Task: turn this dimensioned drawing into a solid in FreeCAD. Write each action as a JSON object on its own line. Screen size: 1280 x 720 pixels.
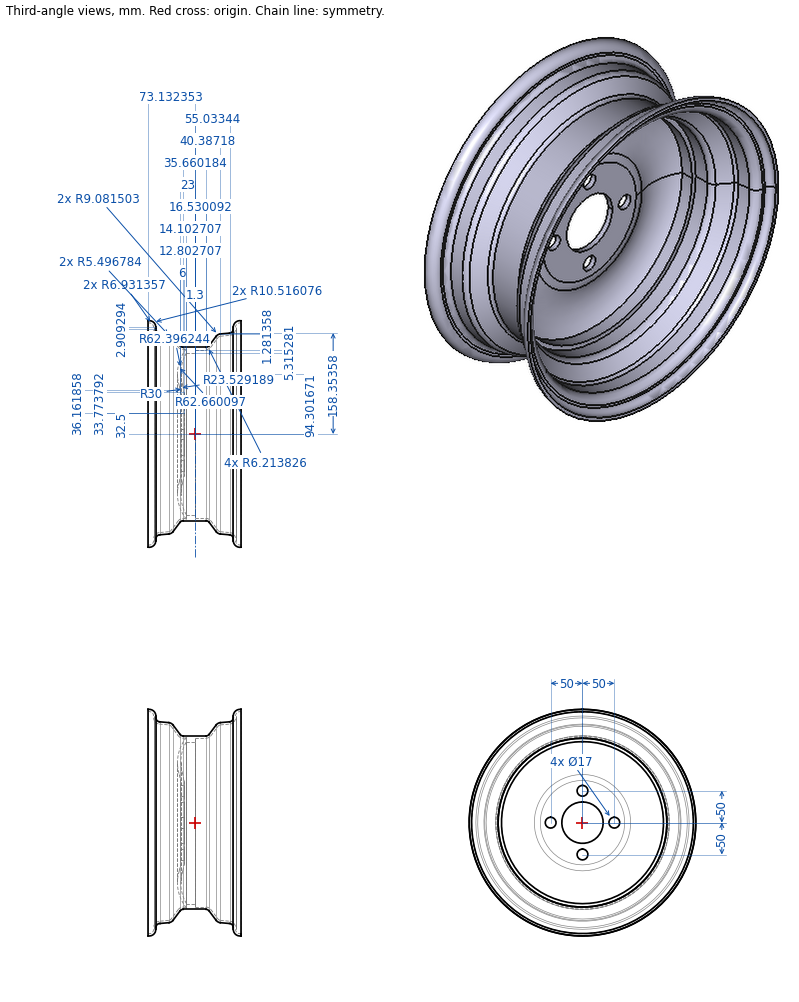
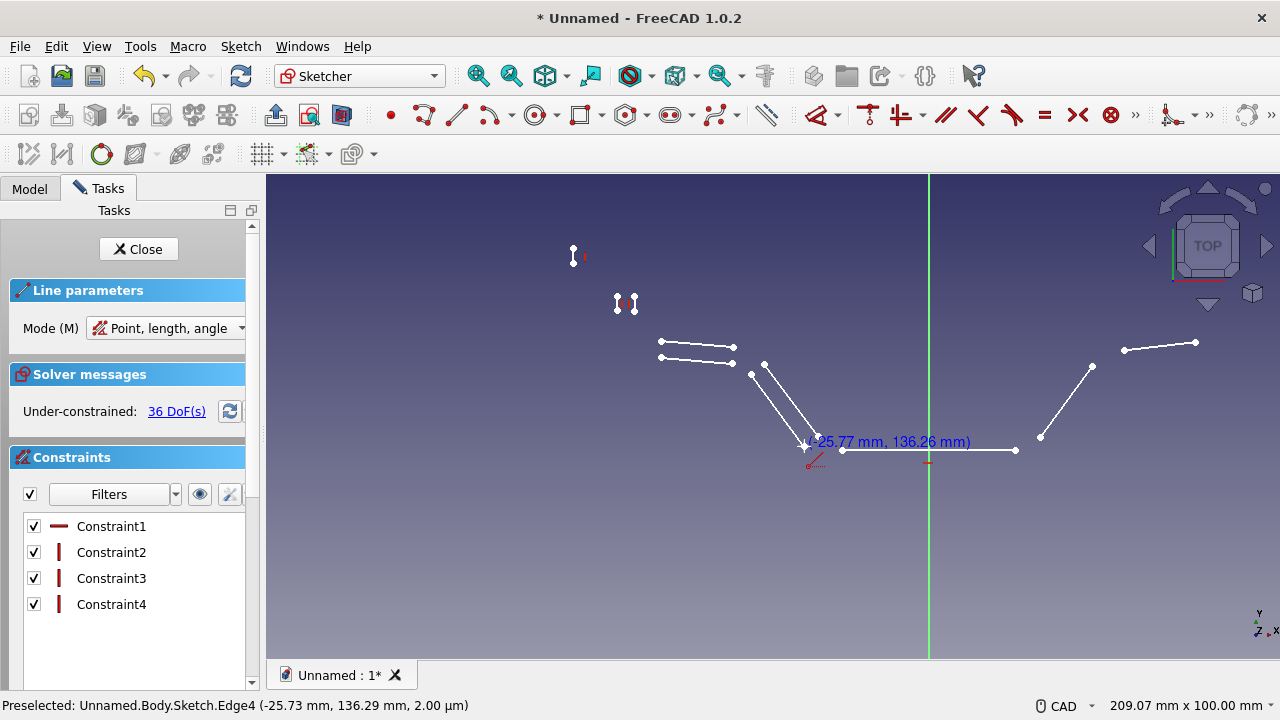
{"action": "key", "text": "g m"}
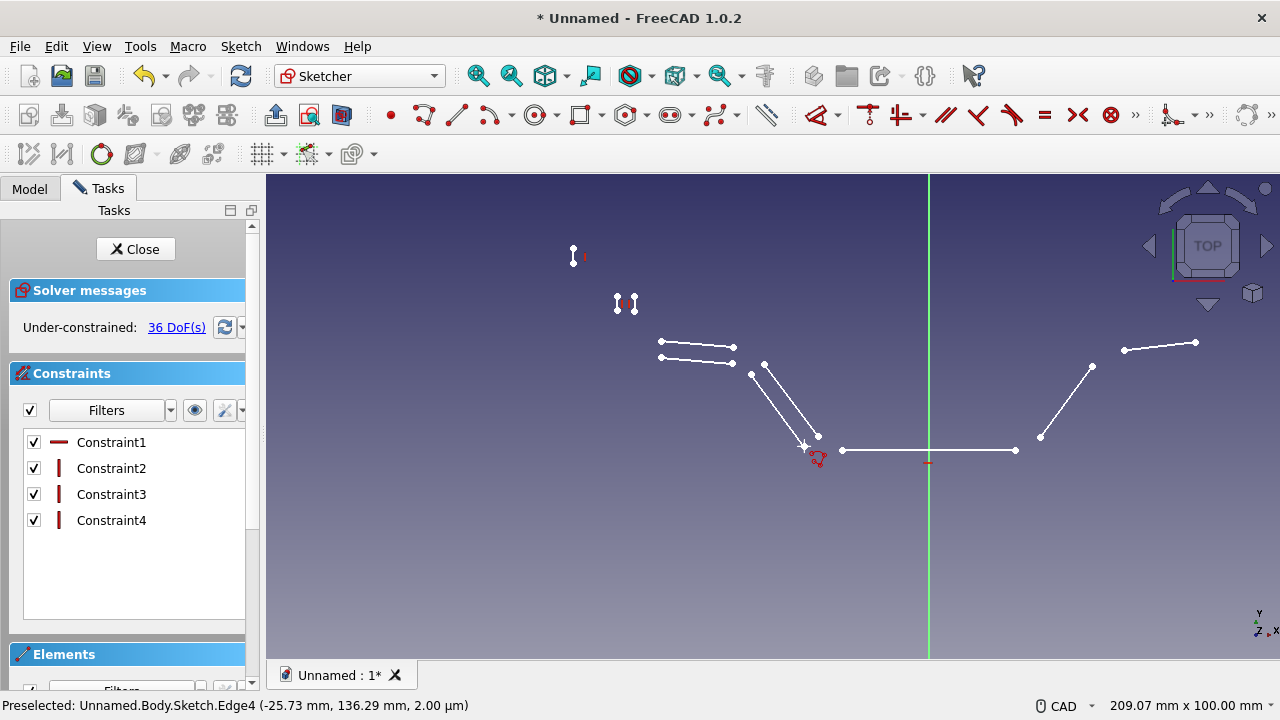
{"action": "scroll", "coordinate": [574, 265], "scroll_direction": "down", "scroll_amount": 5}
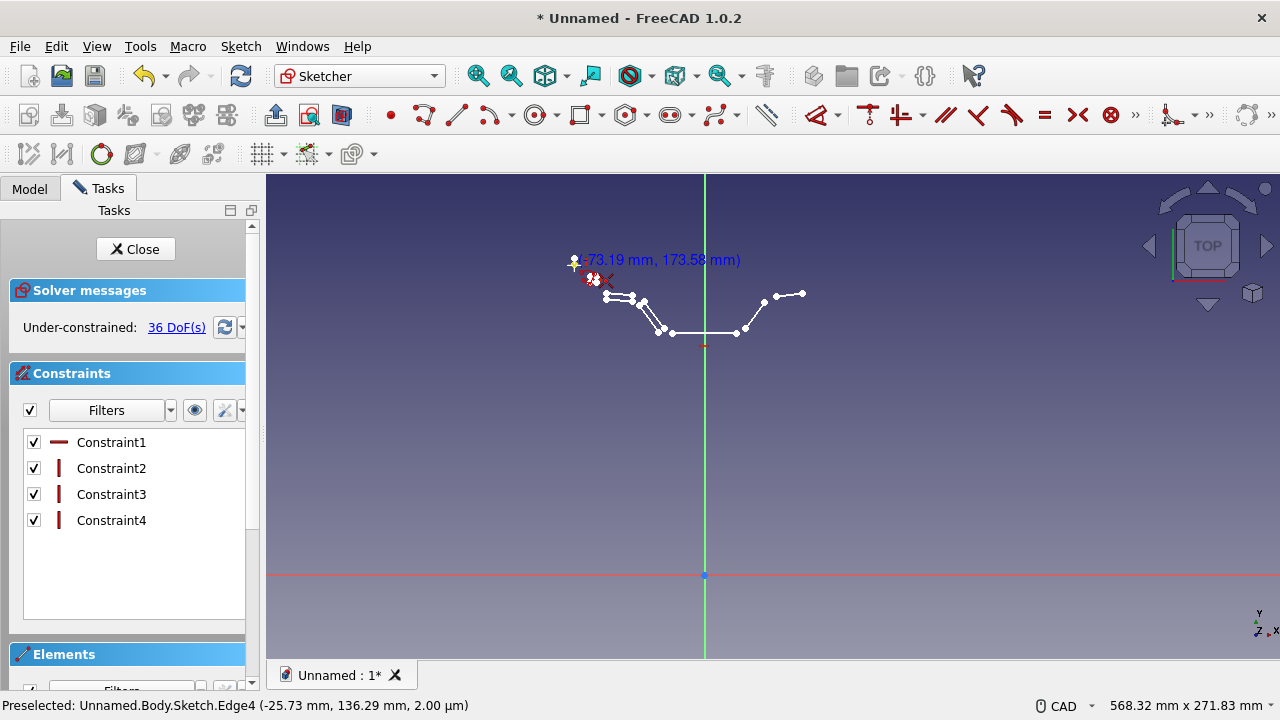
{"action": "left_click", "coordinate": [664, 453]}
{"action": "left_click", "coordinate": [664, 517]}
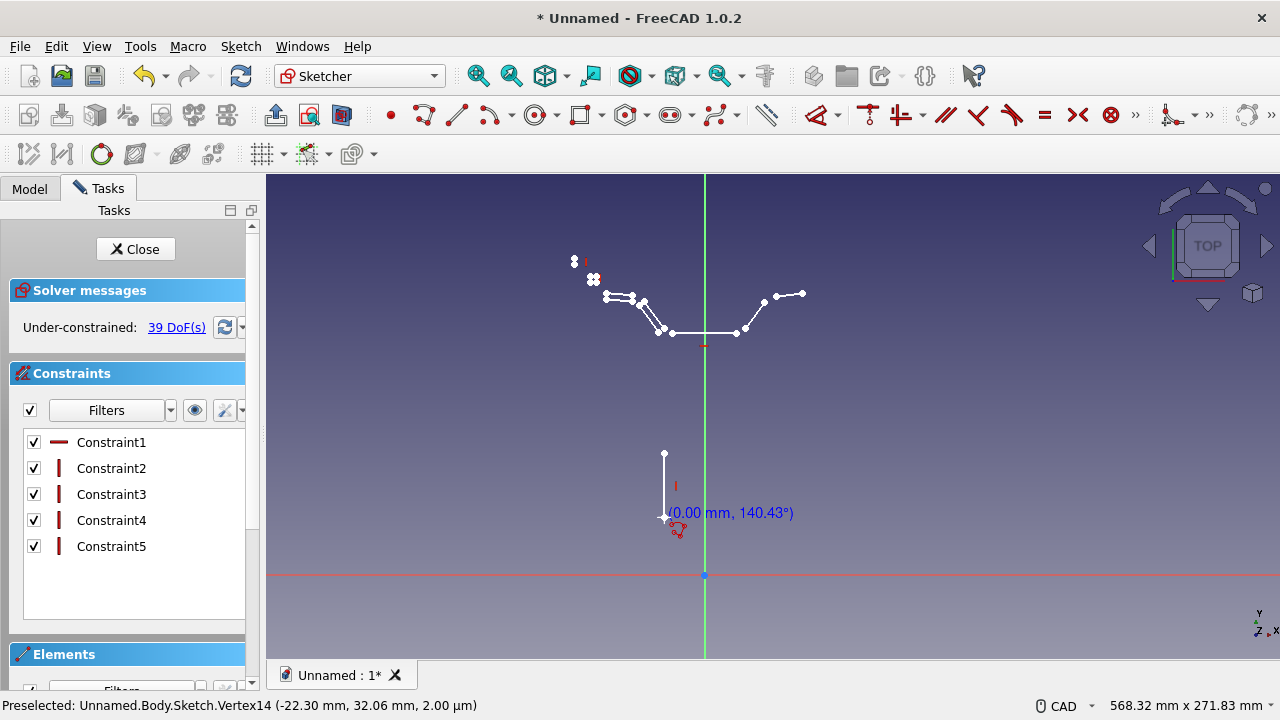
{"action": "scroll", "coordinate": [674, 517], "scroll_direction": "up", "scroll_amount": 2}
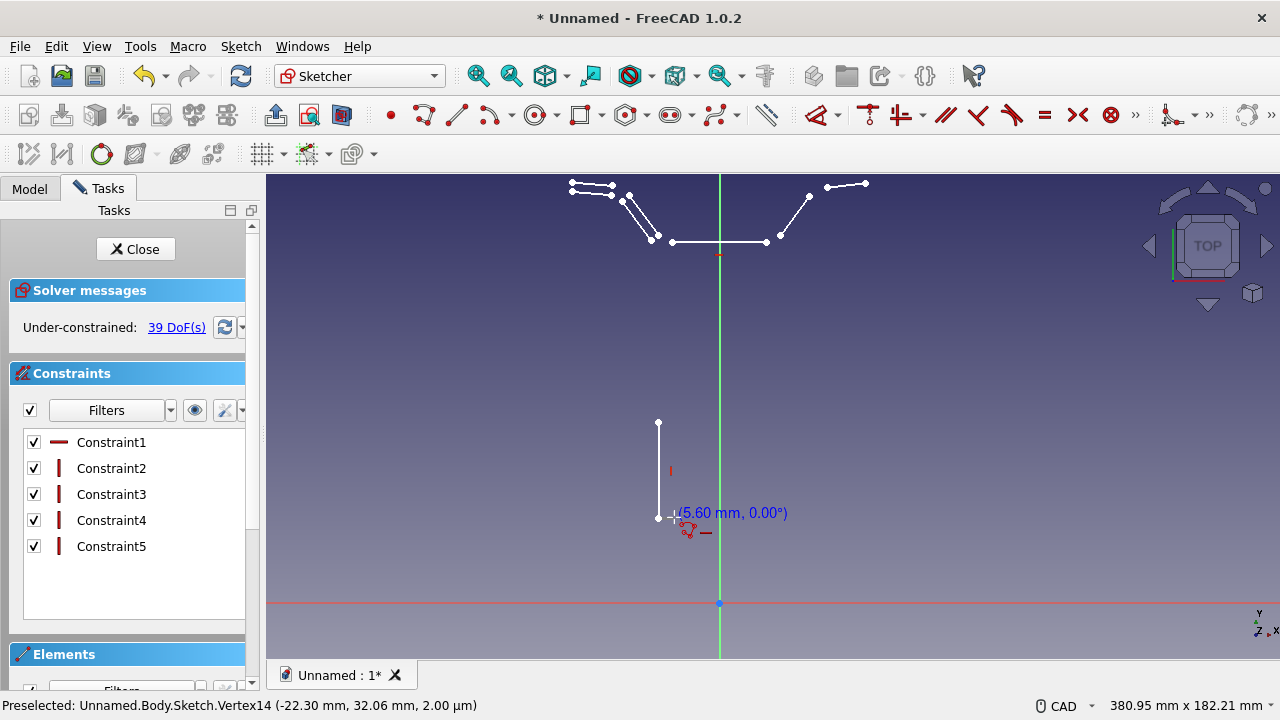
{"action": "left_click", "coordinate": [674, 517]}
{"action": "left_click", "coordinate": [674, 427]}
{"action": "right_click", "coordinate": [674, 427]}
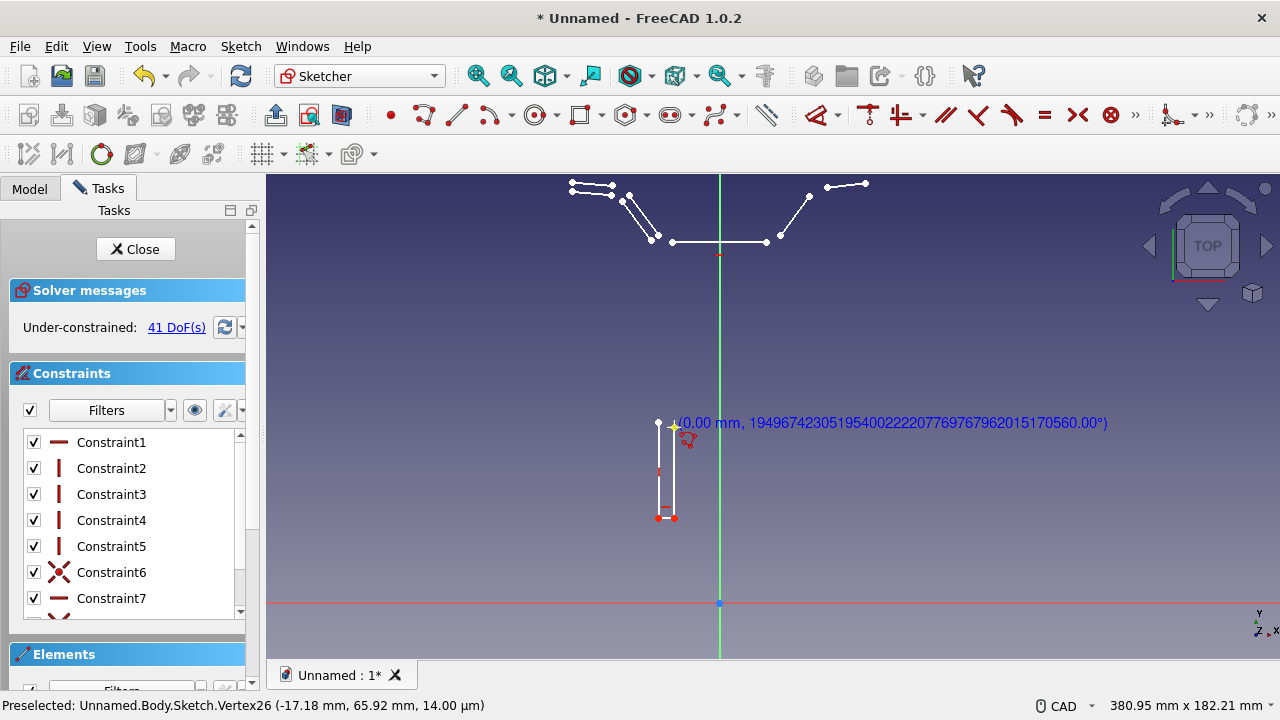
{"action": "left_click", "coordinate": [686, 265]}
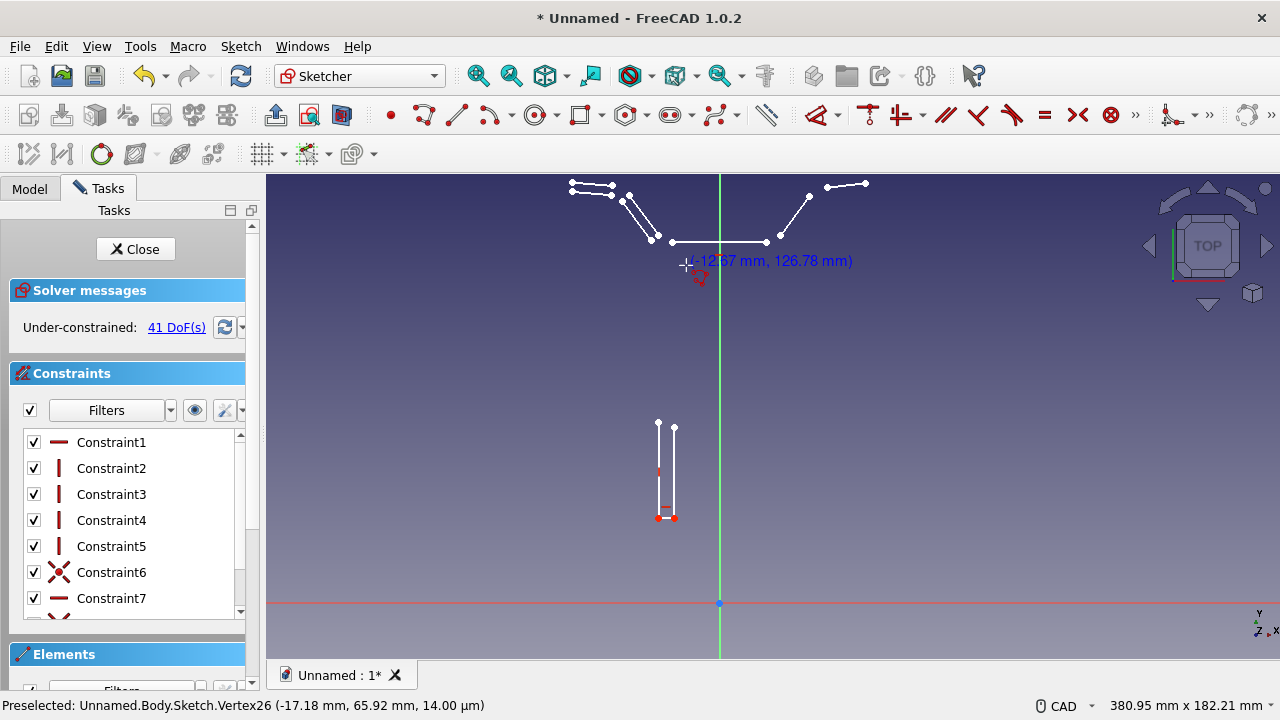
{"action": "scroll", "coordinate": [723, 265], "scroll_direction": "up", "scroll_amount": 8}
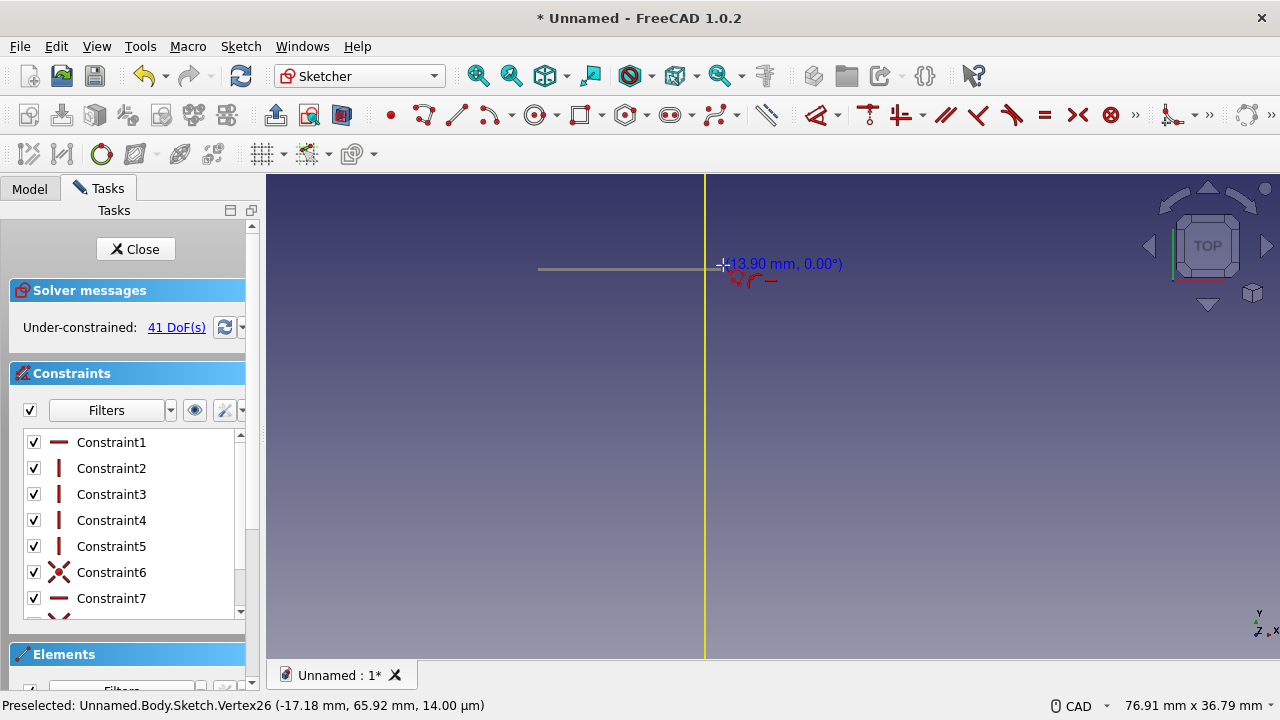
{"action": "left_click", "coordinate": [722, 264]}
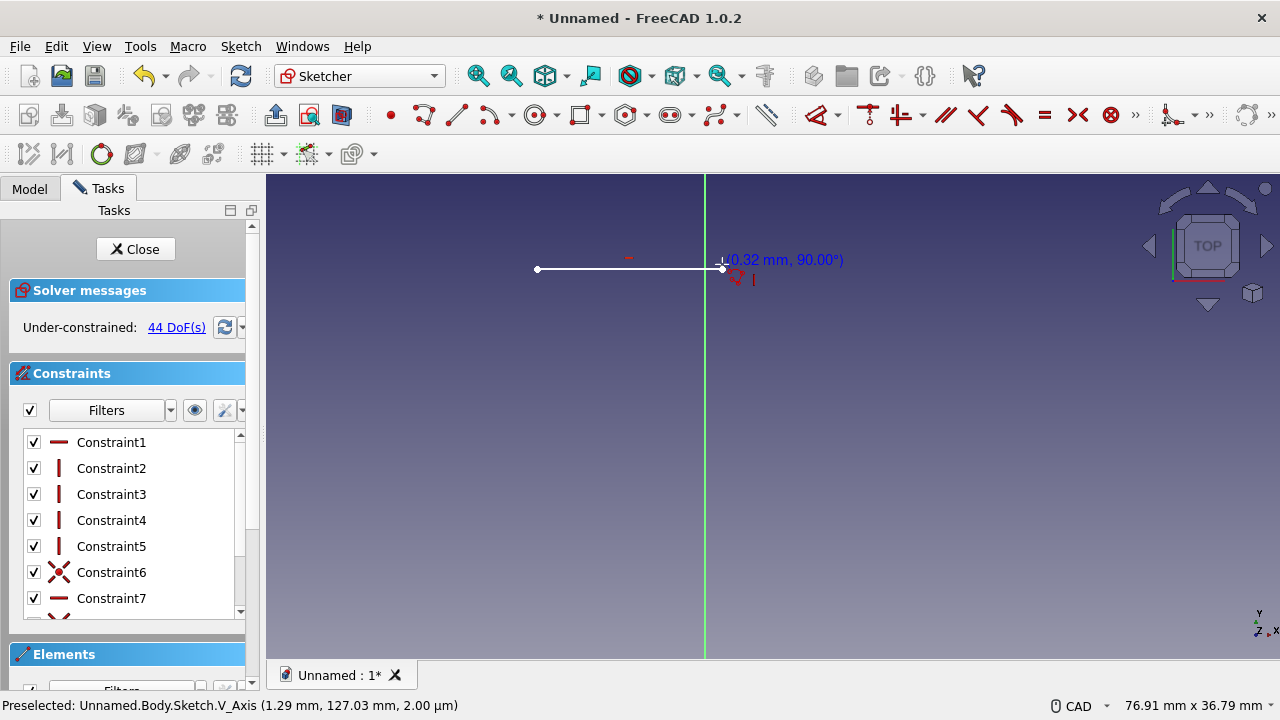
{"action": "scroll", "coordinate": [704, 361], "scroll_direction": "down", "scroll_amount": 10}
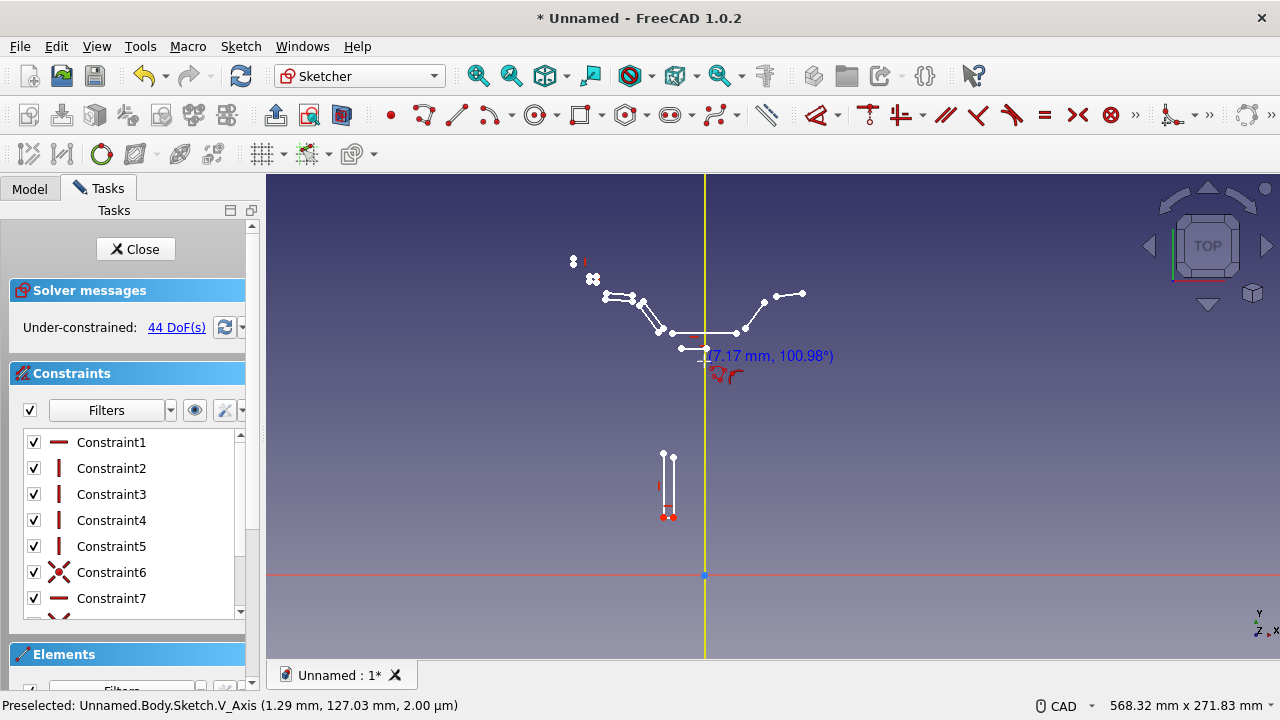
{"action": "scroll", "coordinate": [707, 339], "scroll_direction": "up", "scroll_amount": 10}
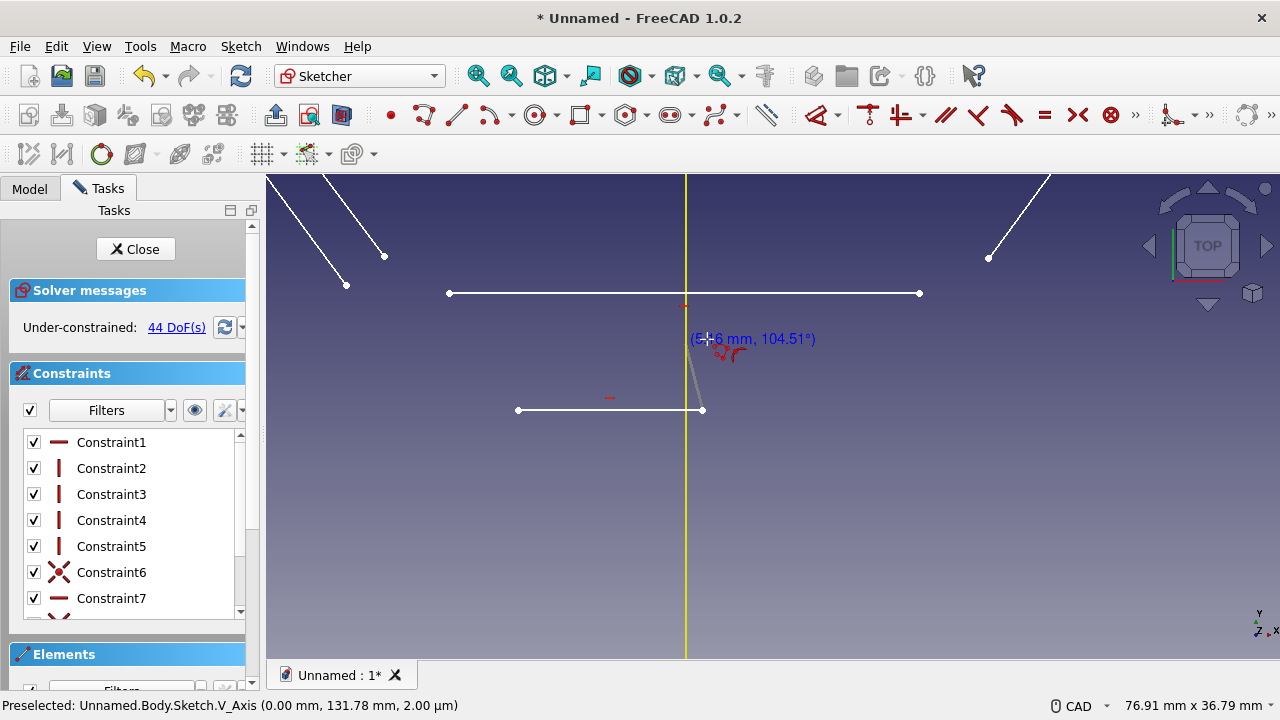
{"action": "left_click", "coordinate": [703, 335]}